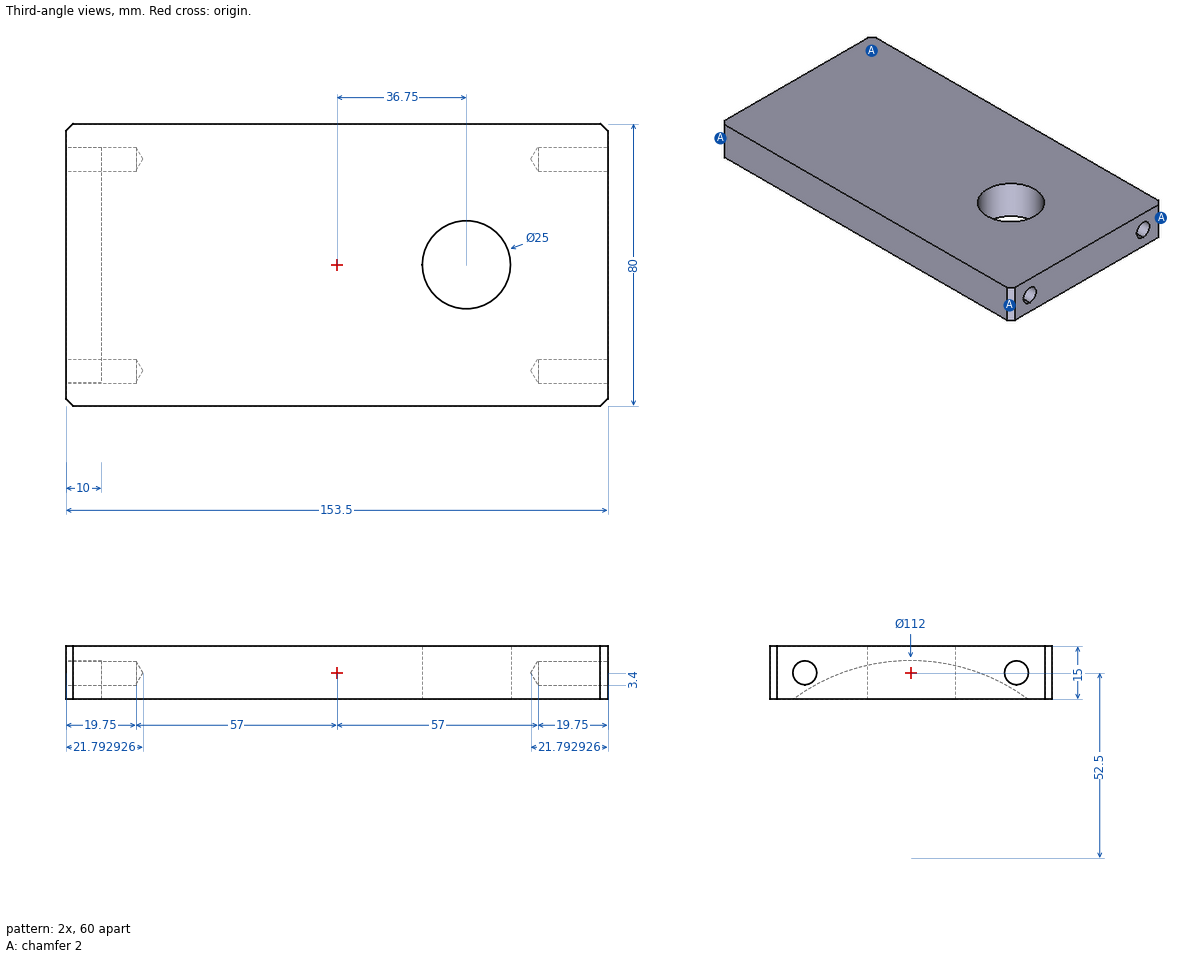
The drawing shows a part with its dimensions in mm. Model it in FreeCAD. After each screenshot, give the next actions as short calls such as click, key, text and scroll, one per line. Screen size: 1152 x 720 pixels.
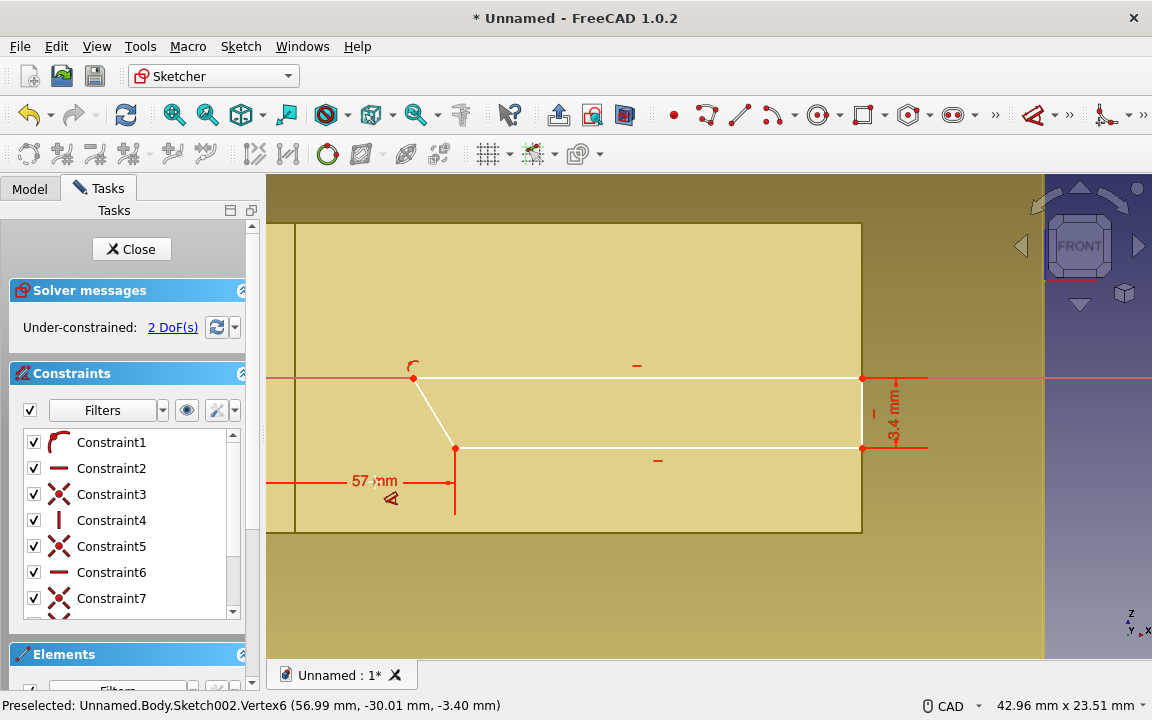
click(740, 448)
click(659, 482)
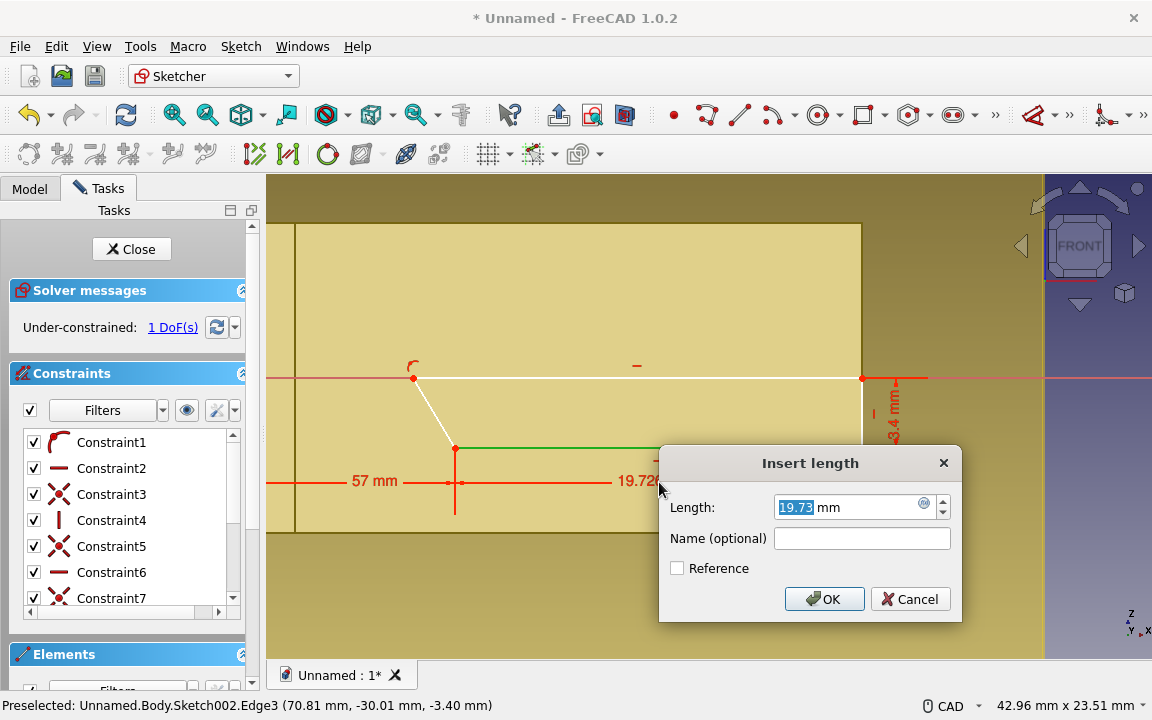
text(19.75)
key(Return)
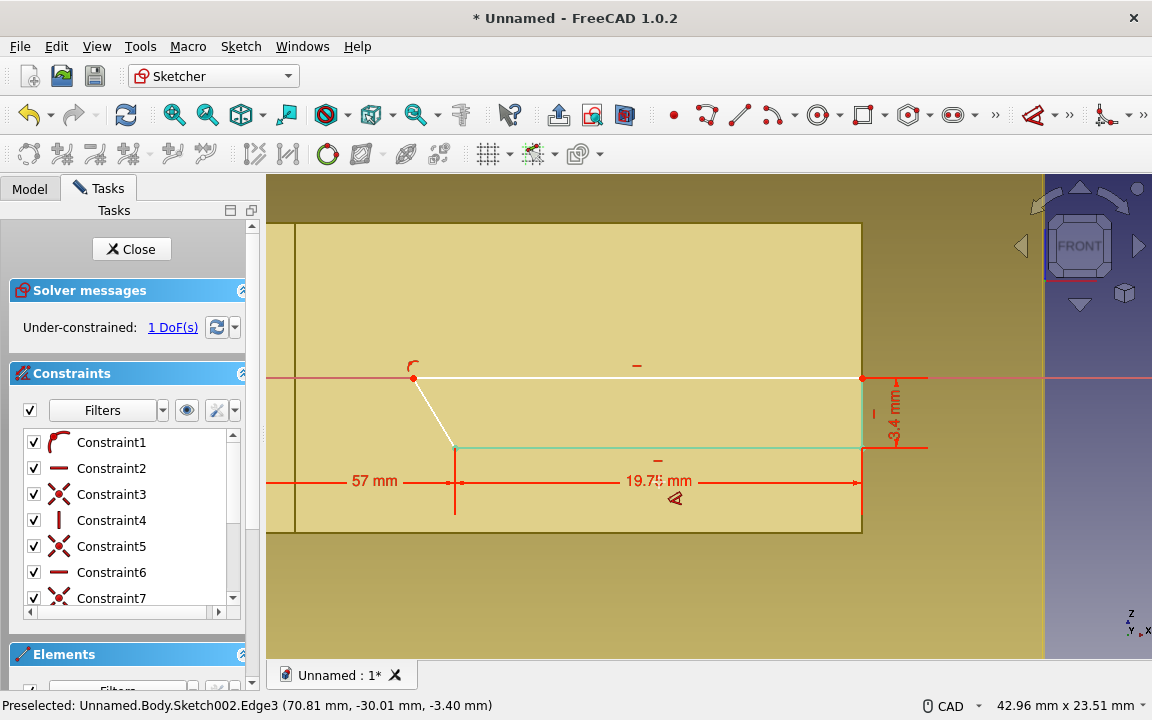
click(548, 378)
click(638, 344)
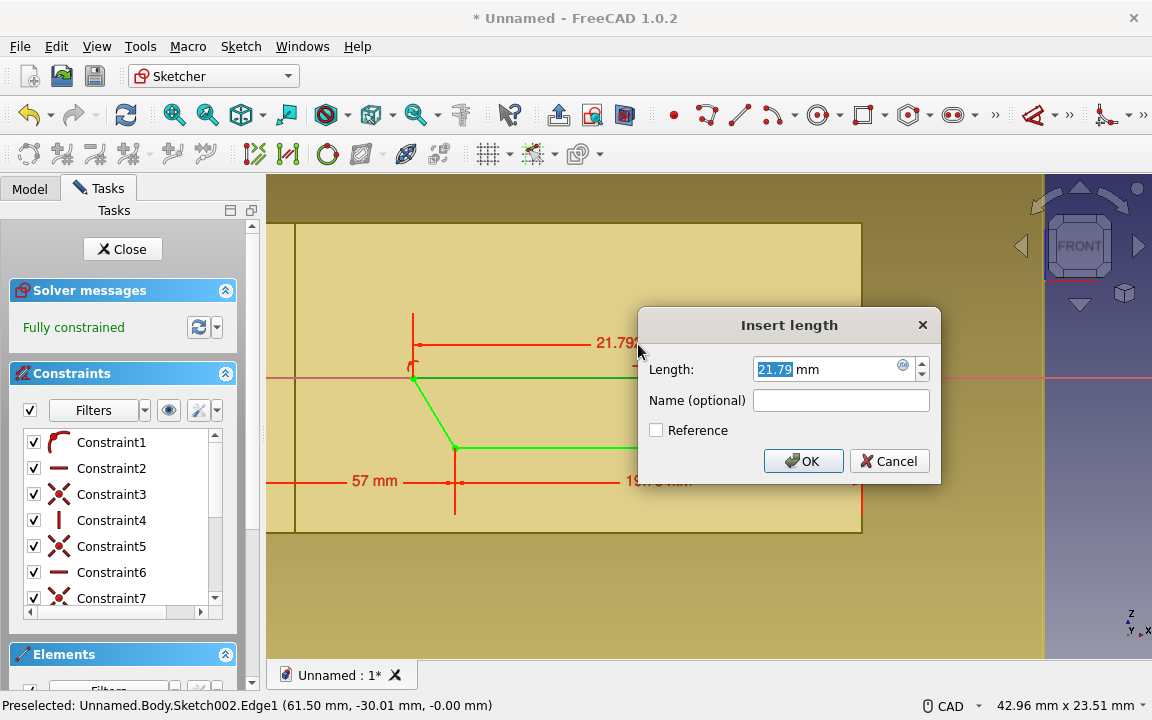
text(21.792926)
key(Return)
key(Escape)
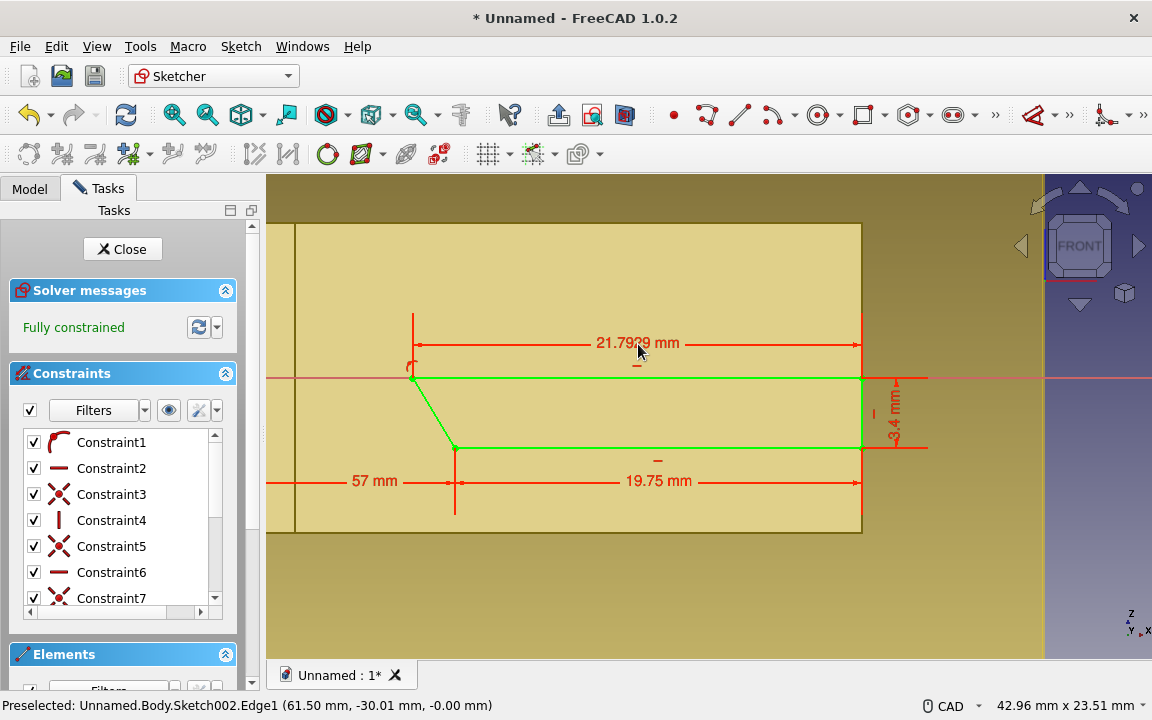
click(123, 249)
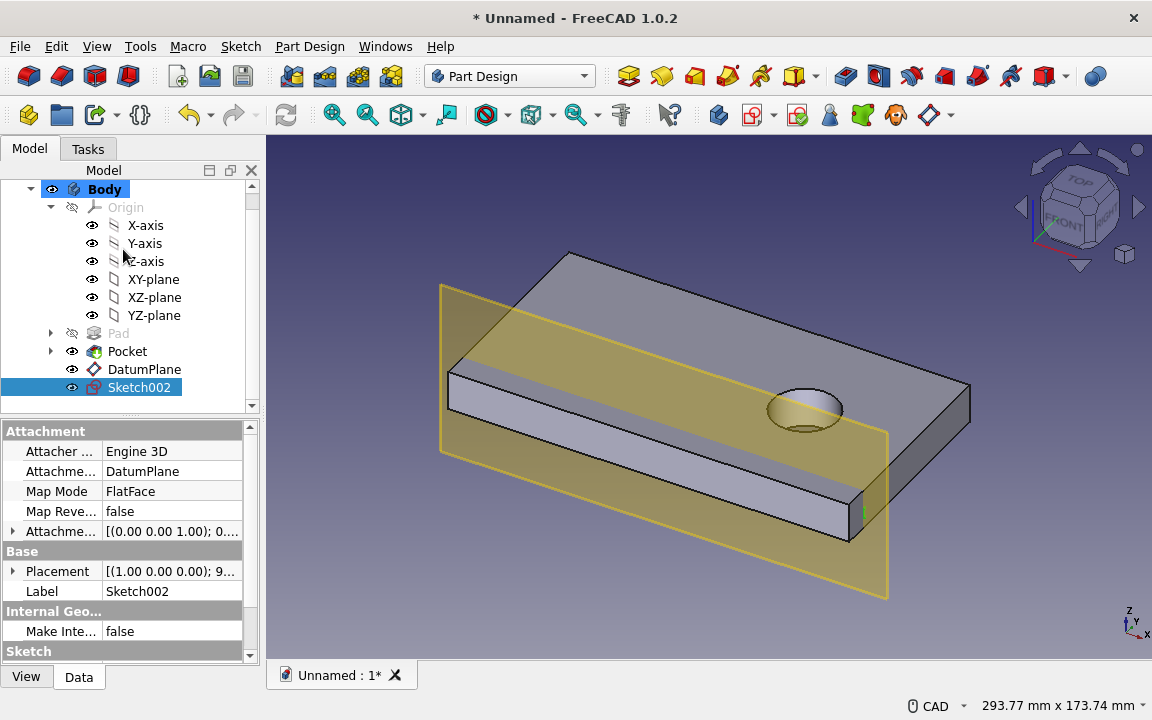
click(912, 76)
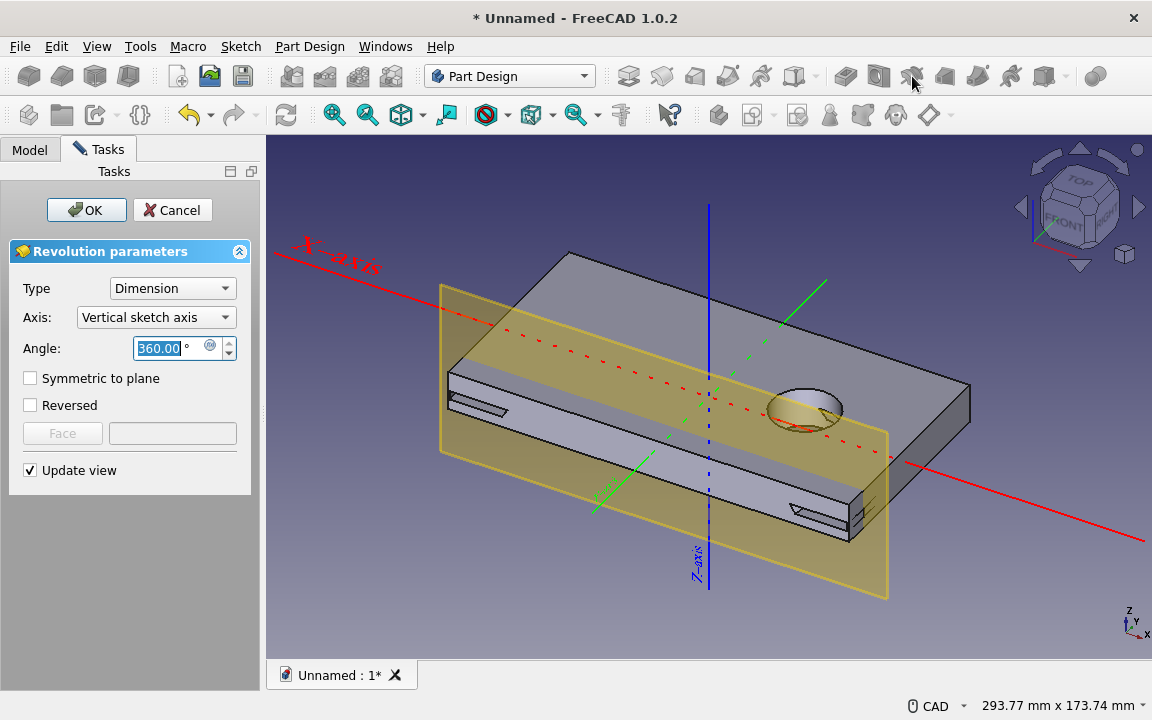
click(157, 318)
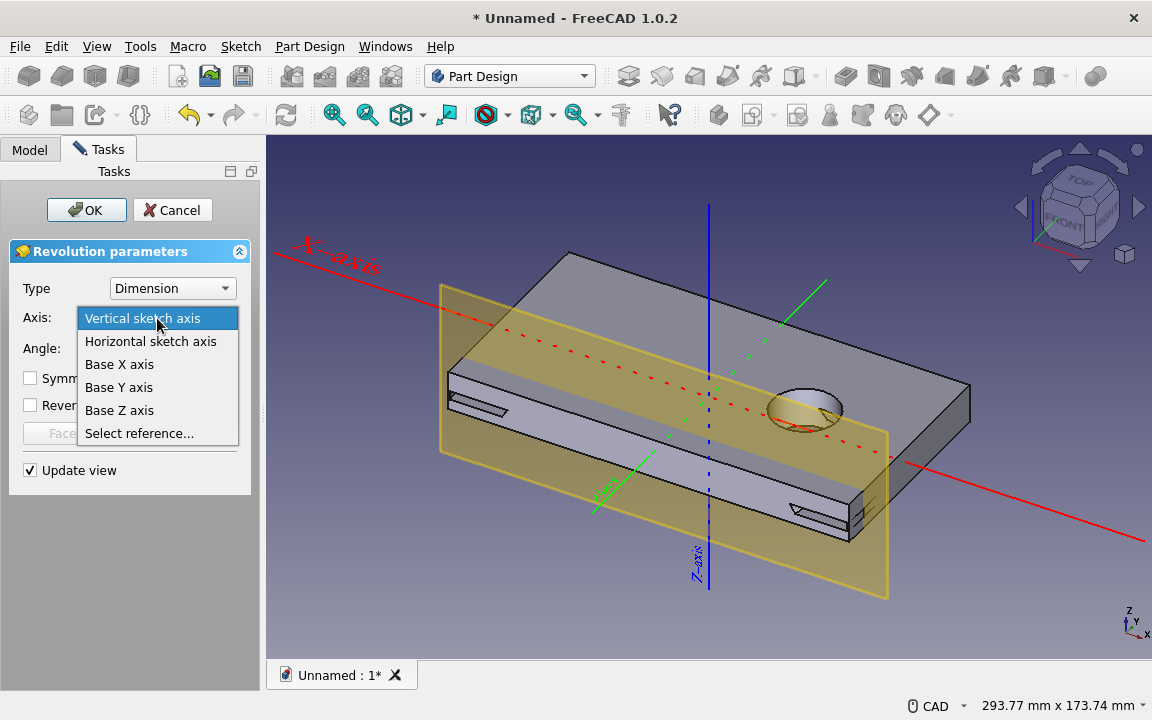
click(156, 342)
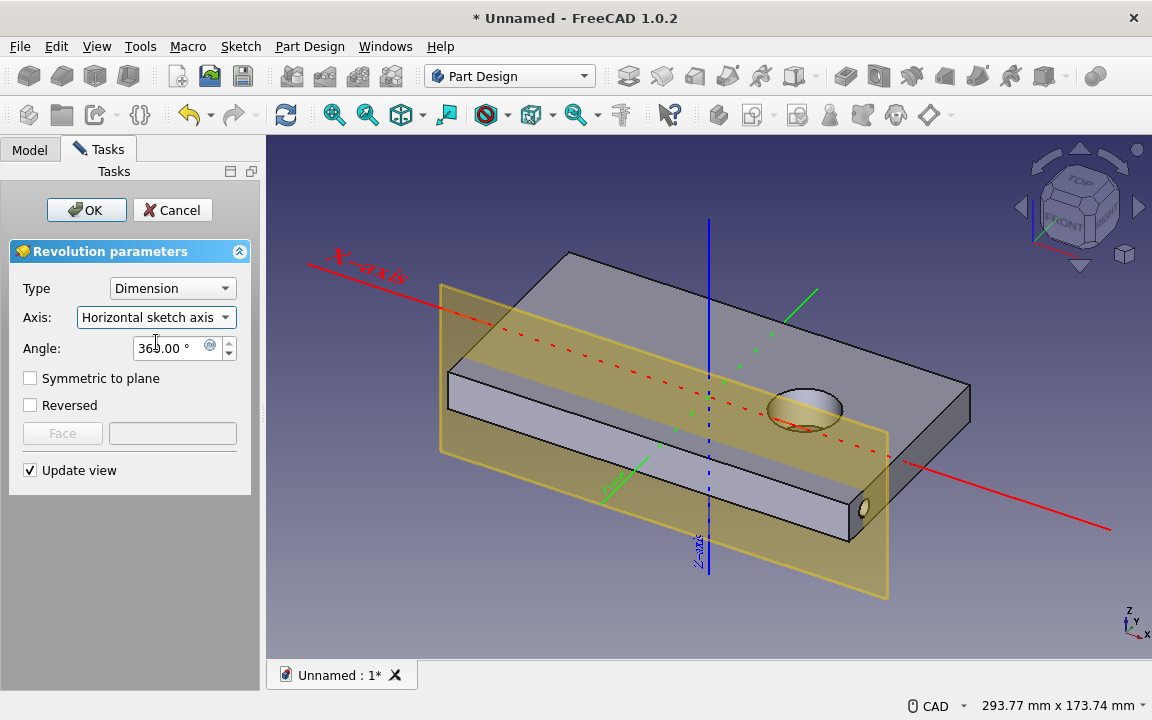
click(87, 210)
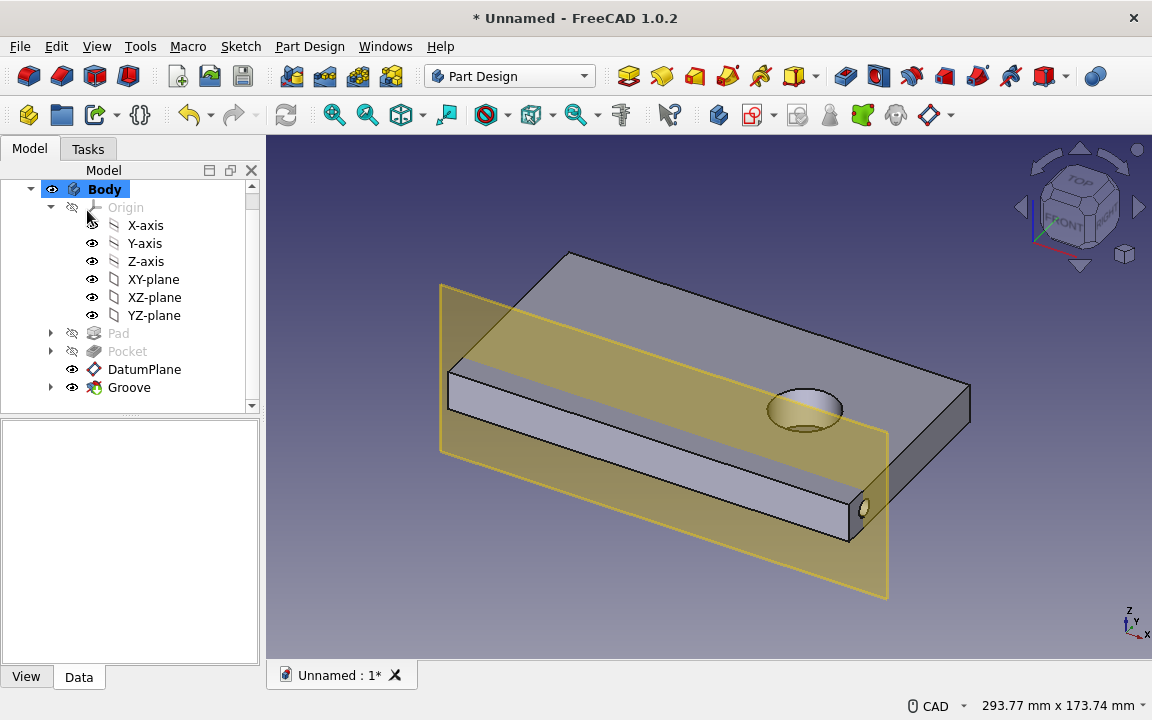
click(117, 369)
key(space)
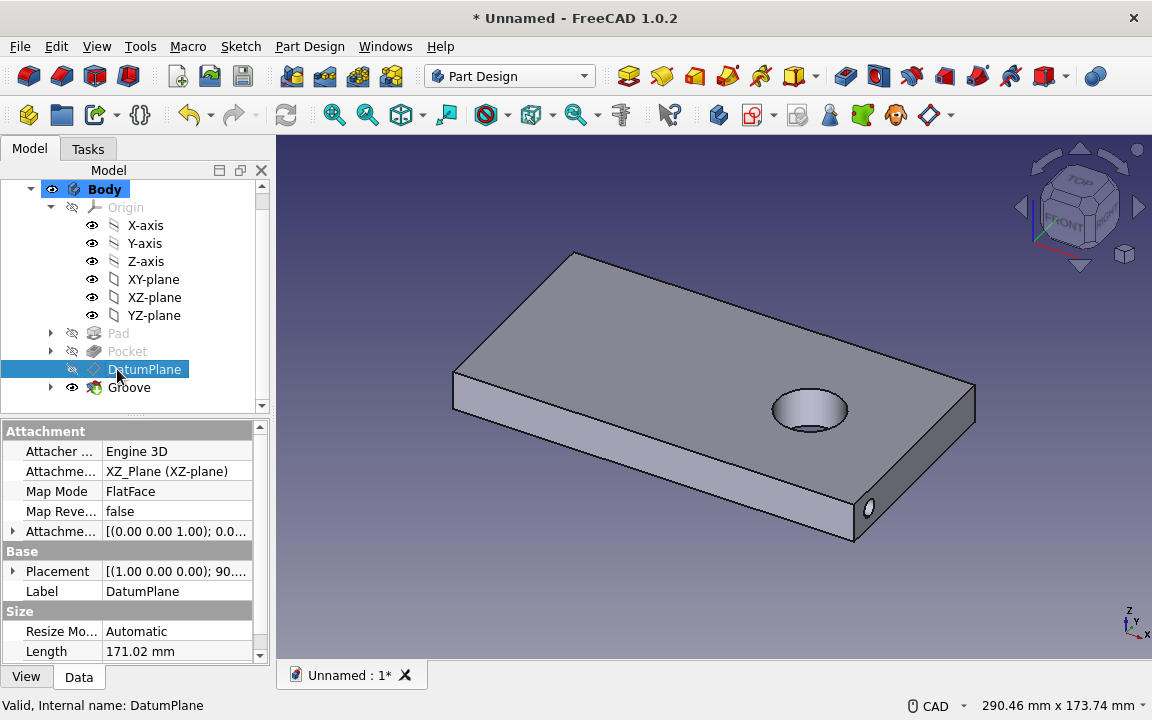
click(117, 387)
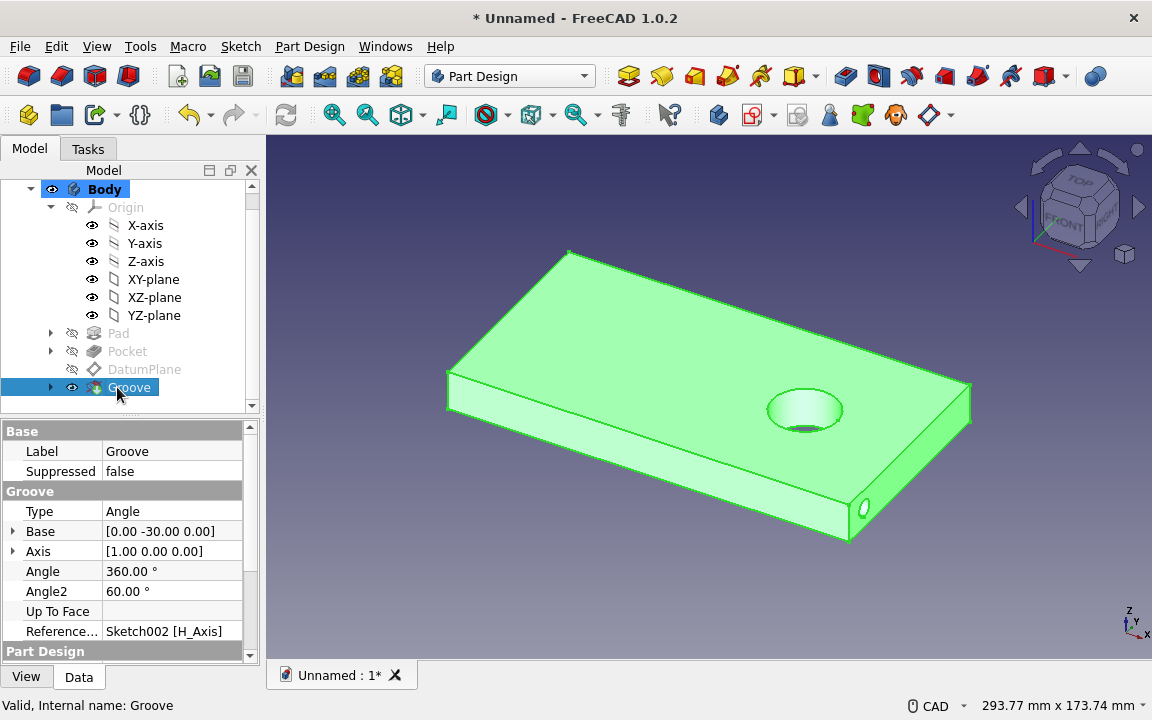
click(325, 76)